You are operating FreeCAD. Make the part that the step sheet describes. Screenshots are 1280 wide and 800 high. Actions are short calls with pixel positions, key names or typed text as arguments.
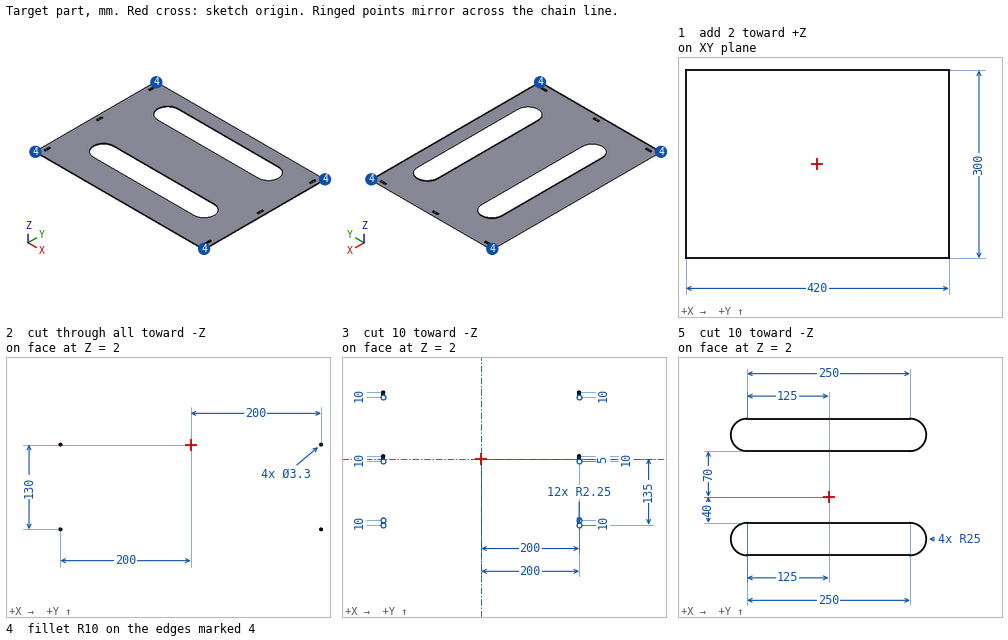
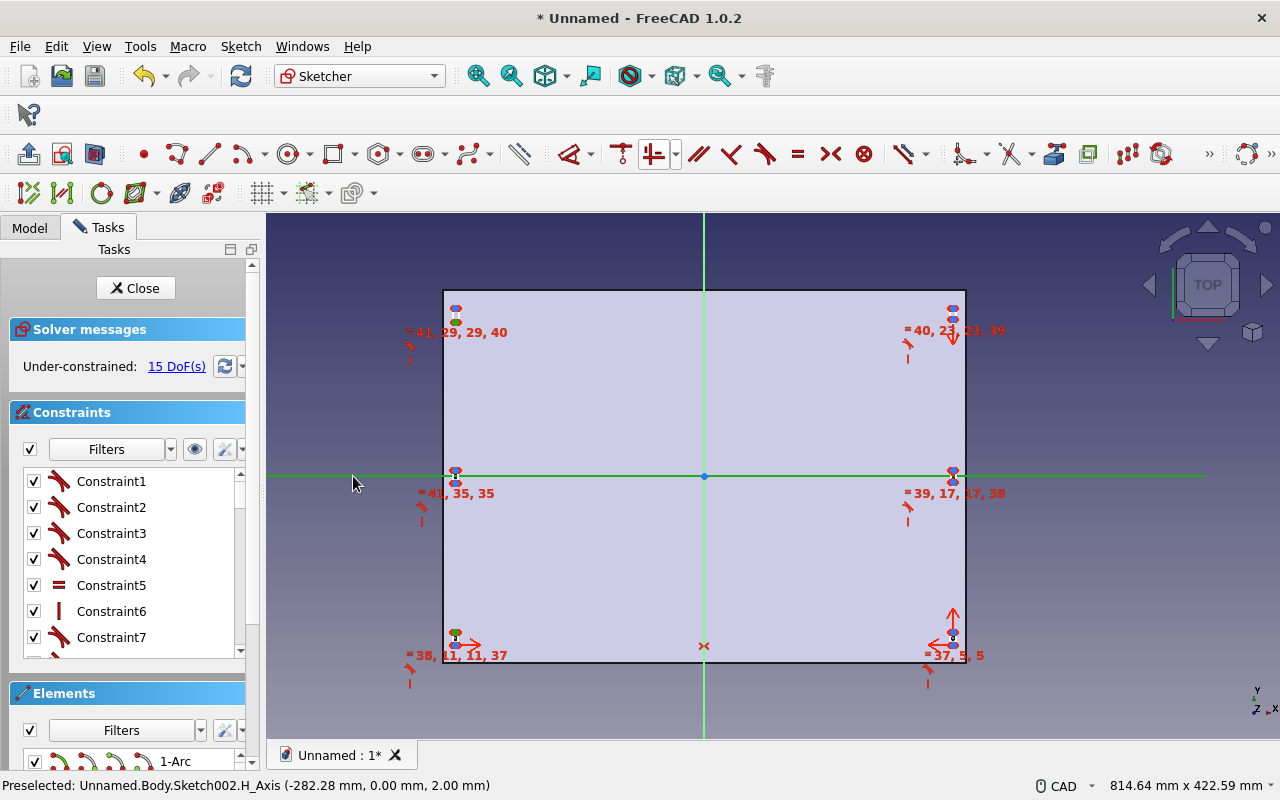
key(s)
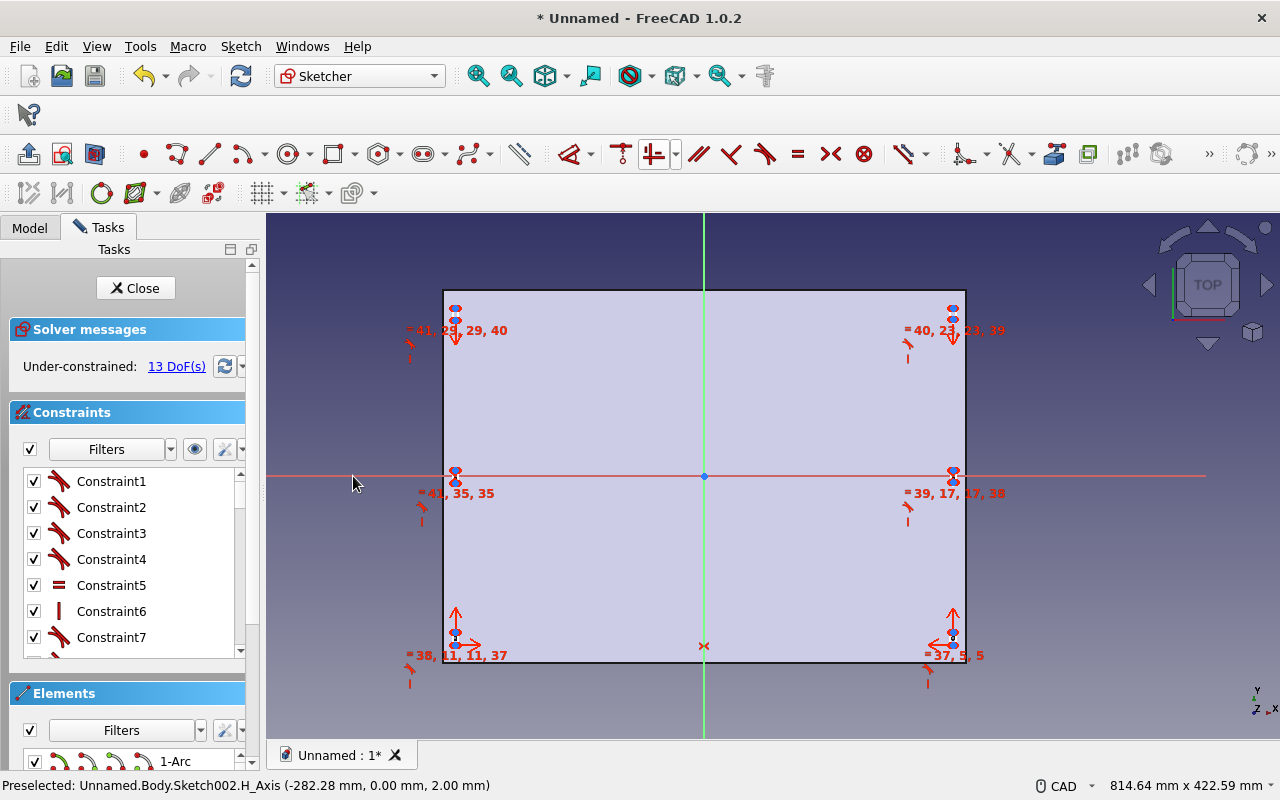
scroll(953, 483, up, 8)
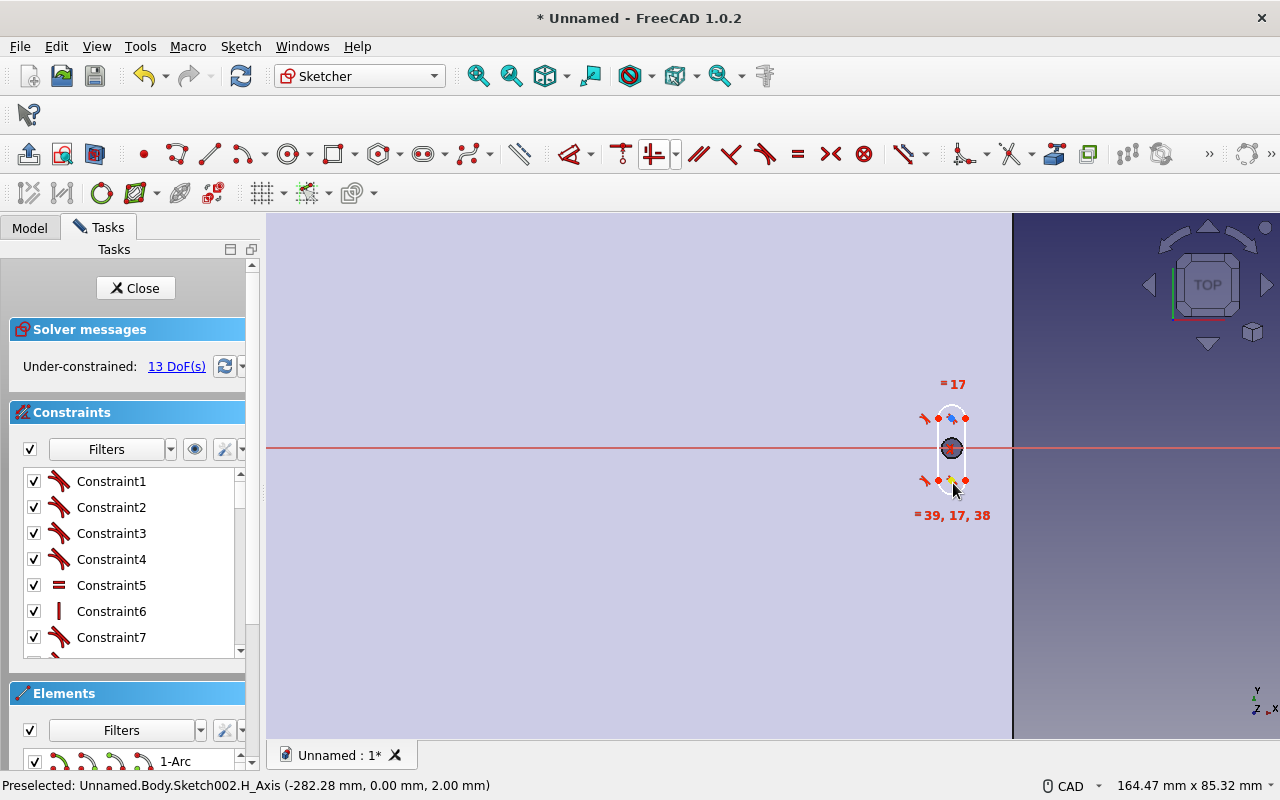
click(952, 481)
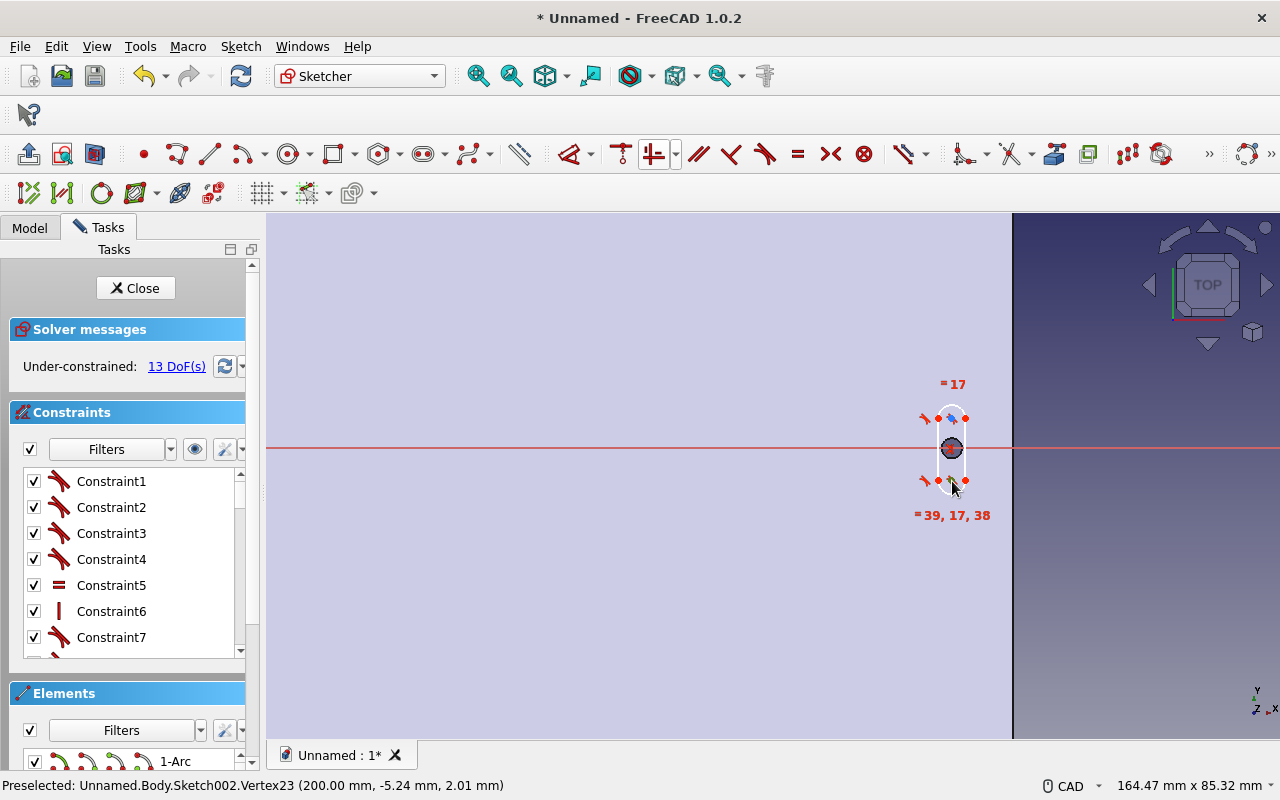
scroll(954, 483, down, 8)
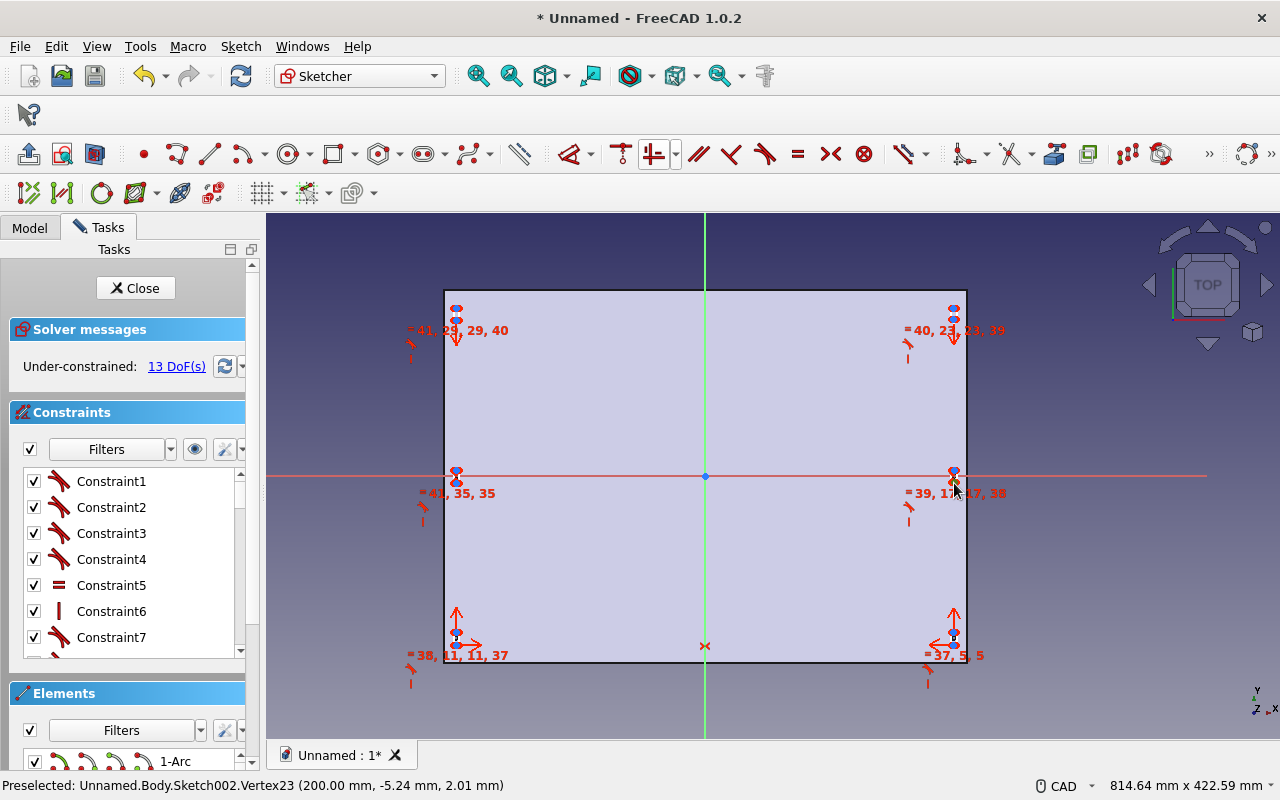
scroll(456, 483, up, 8)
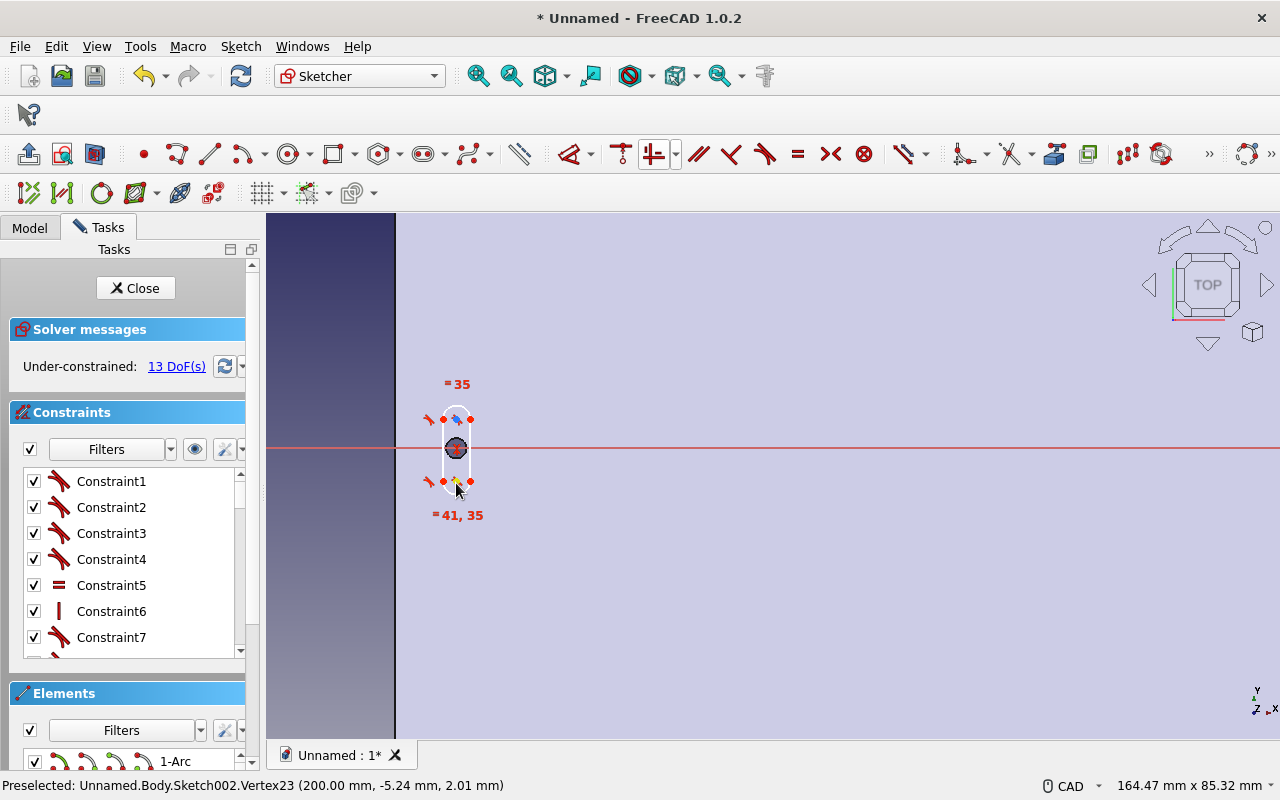
click(457, 481)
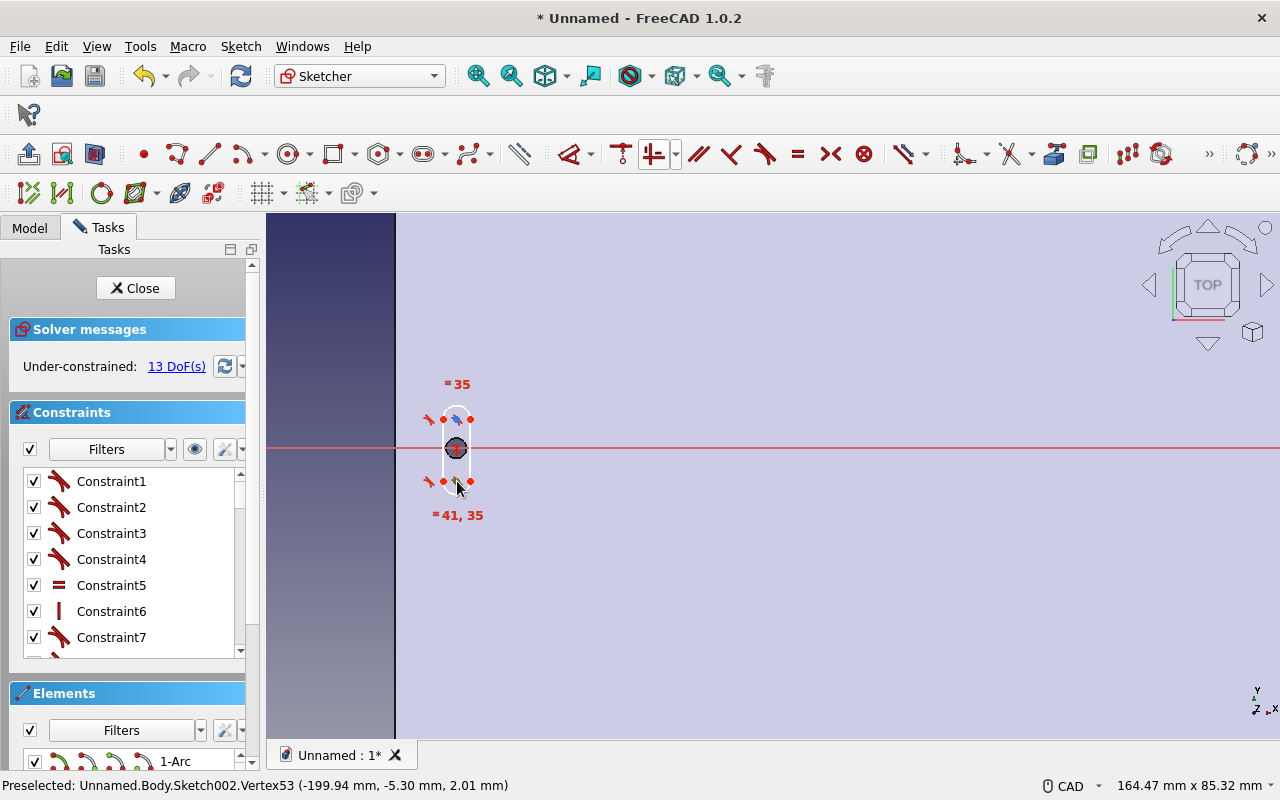
scroll(455, 483, down, 8)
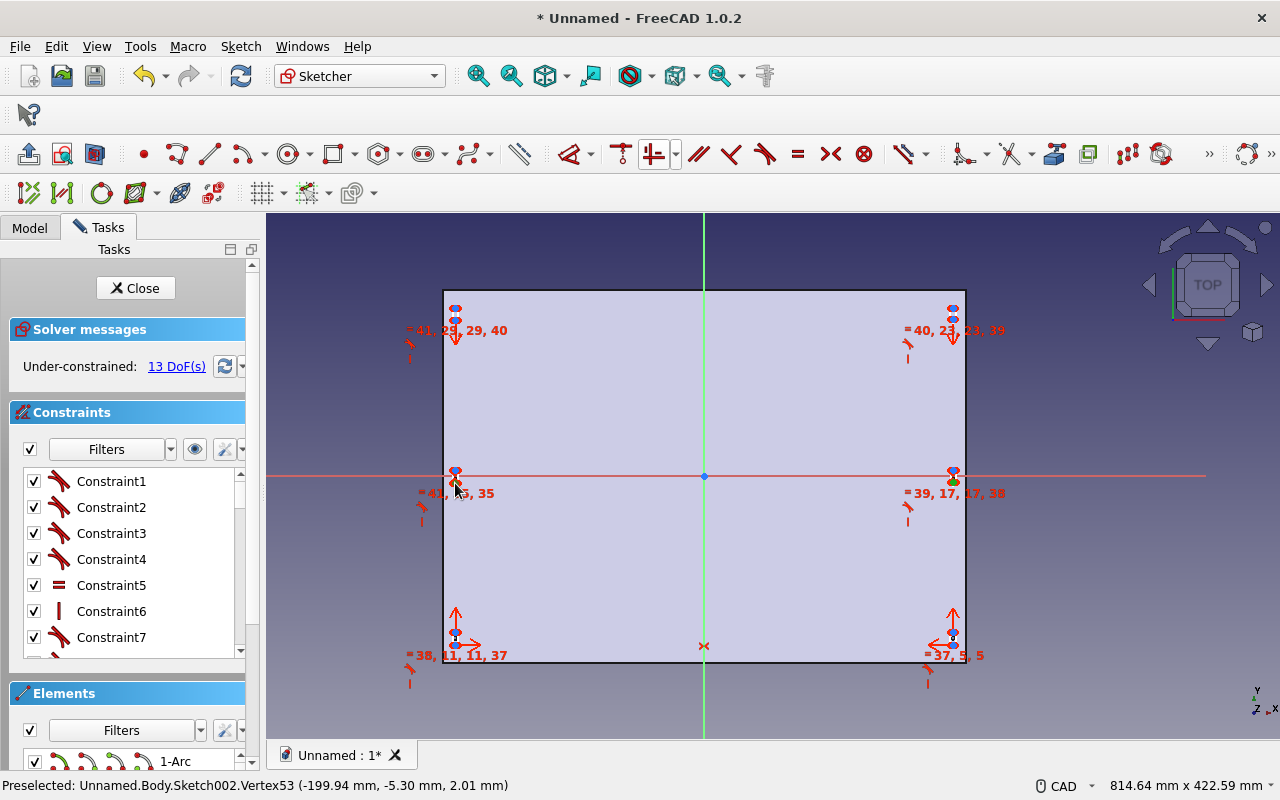
click(704, 677)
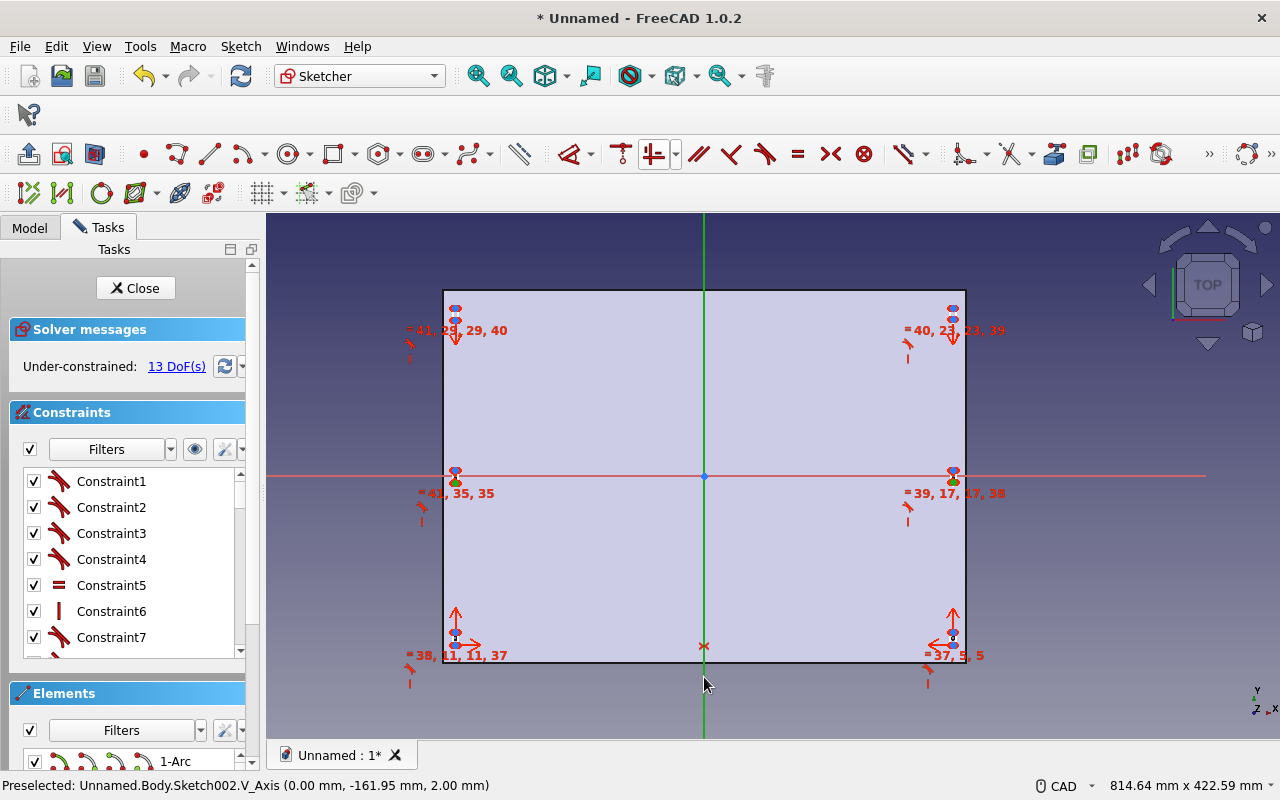
key(s)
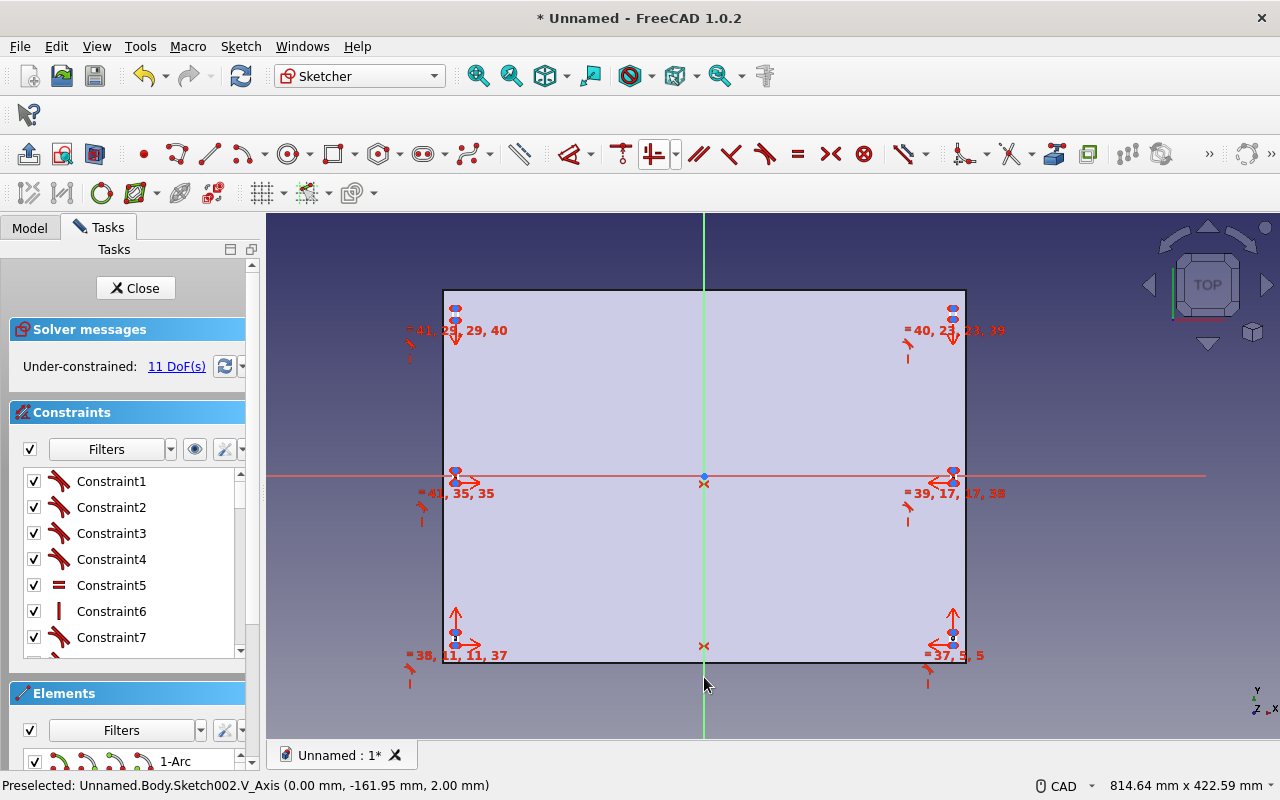
click(568, 154)